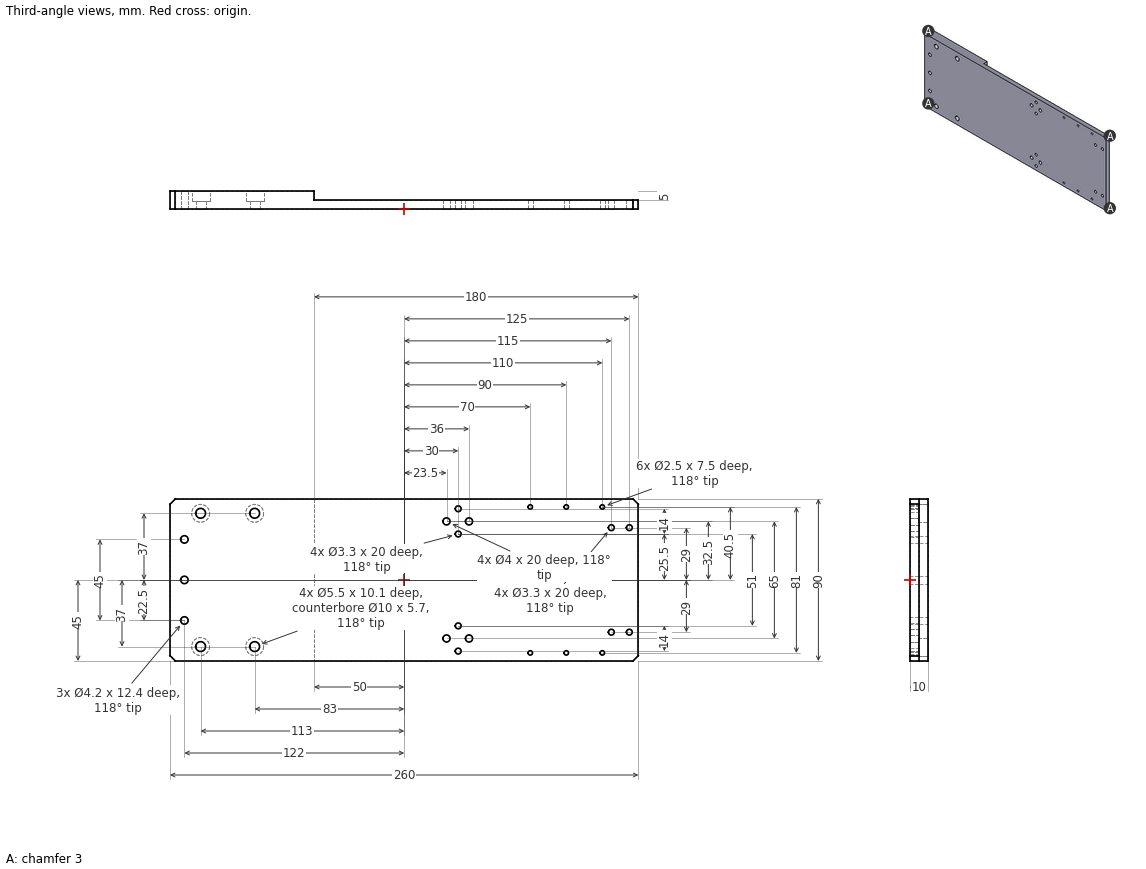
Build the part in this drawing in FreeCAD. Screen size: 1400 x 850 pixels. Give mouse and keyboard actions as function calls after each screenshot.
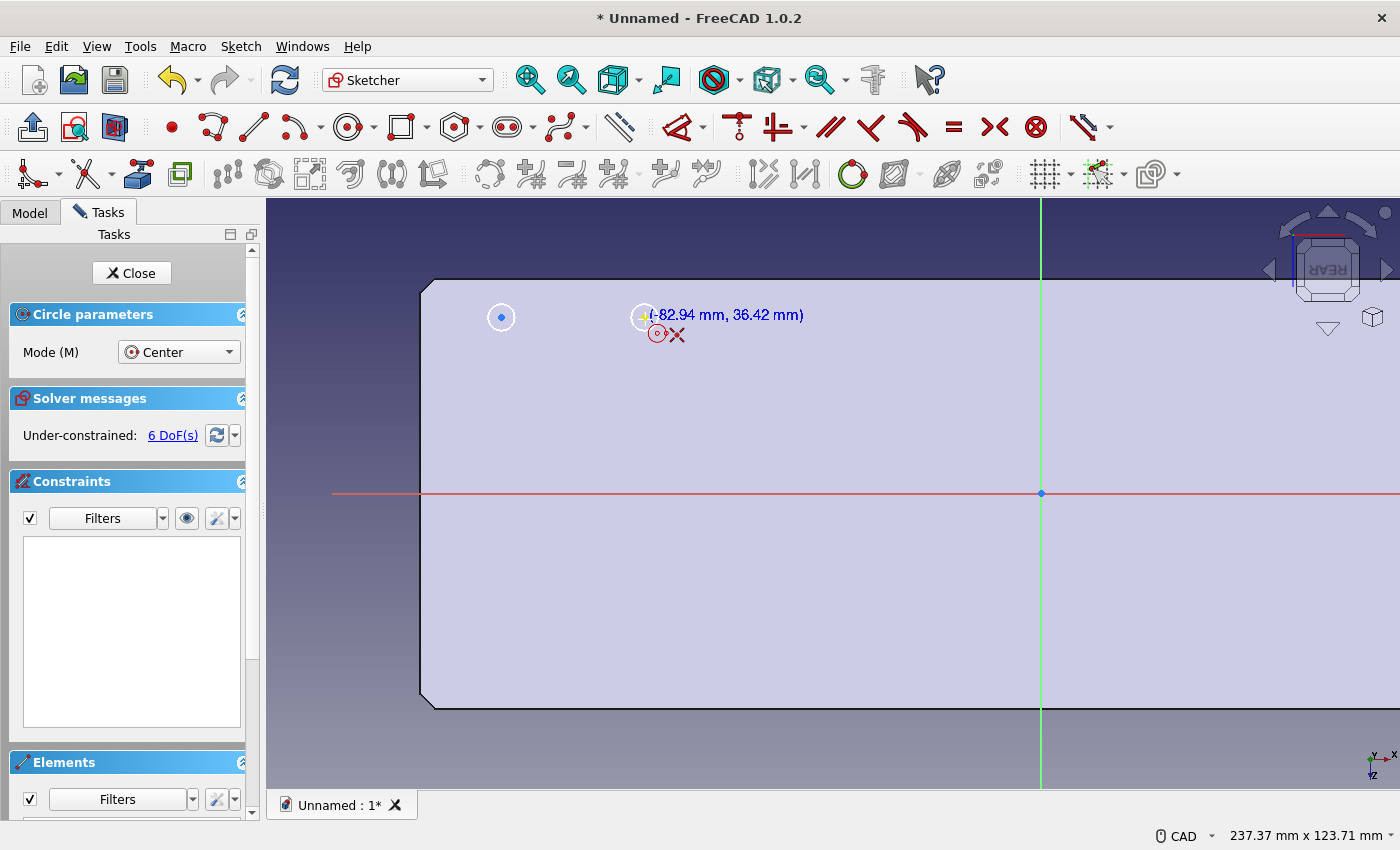
scroll(645, 670, up, 3)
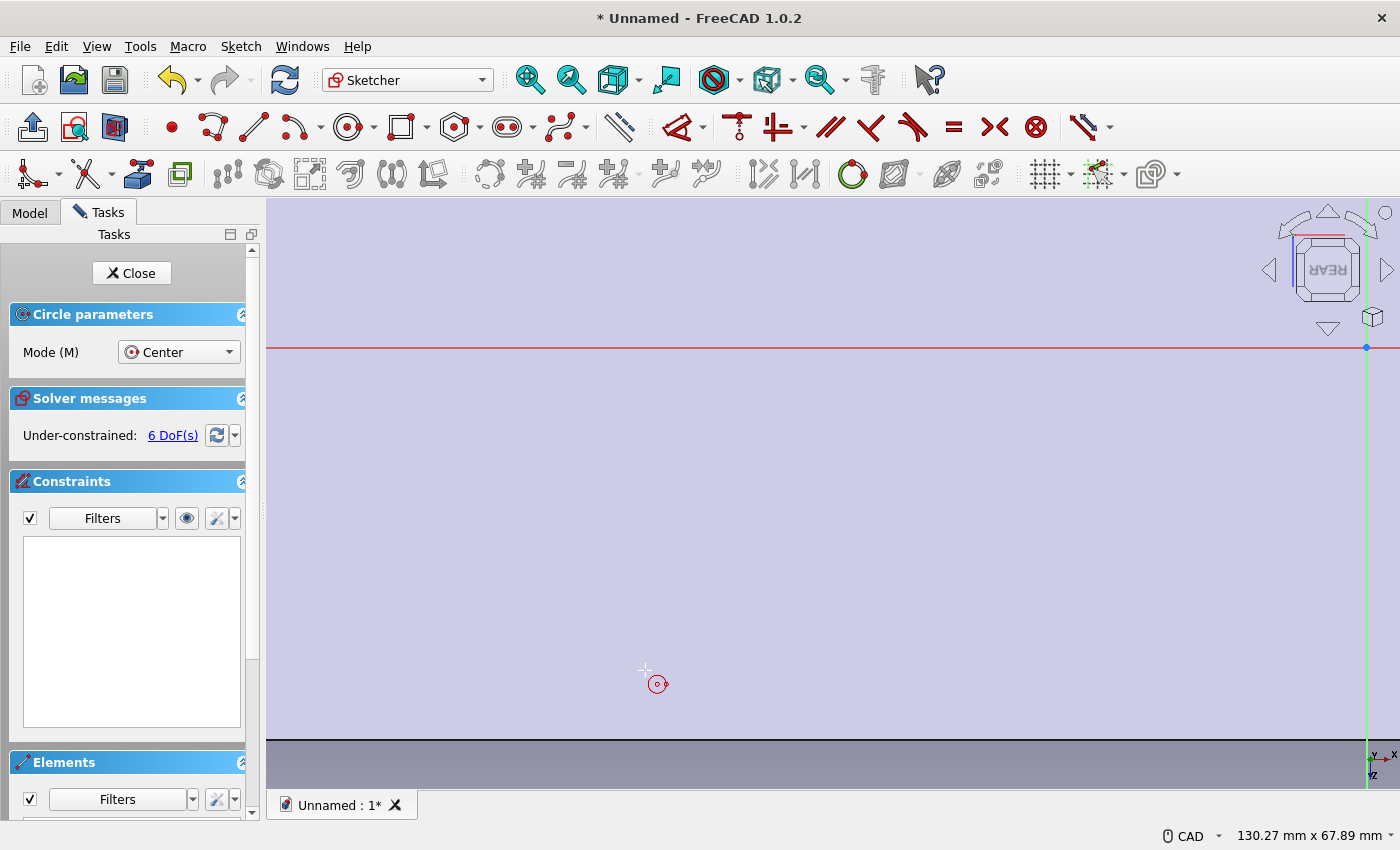
click(644, 670)
click(661, 653)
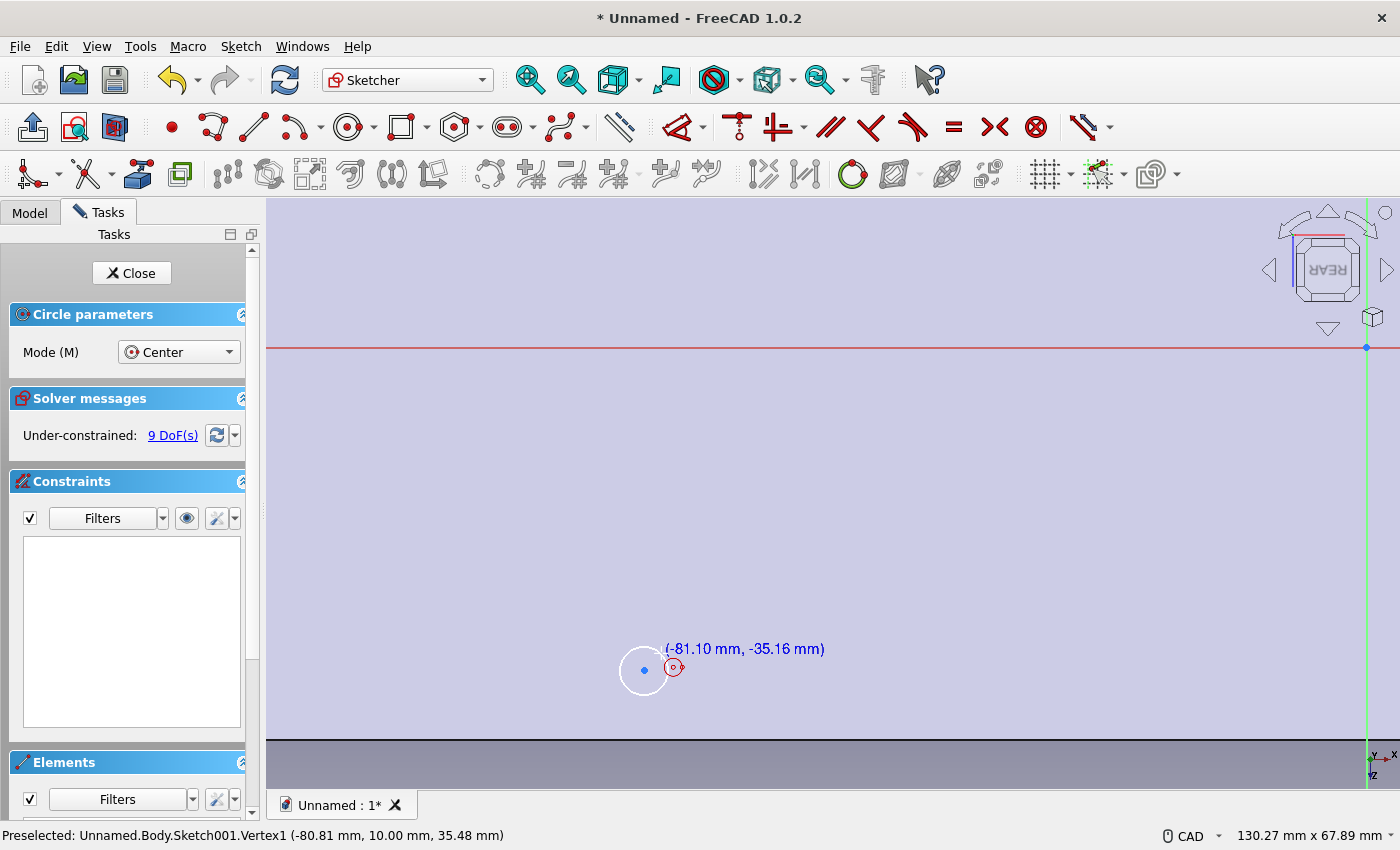
click(383, 670)
click(400, 653)
key(Escape)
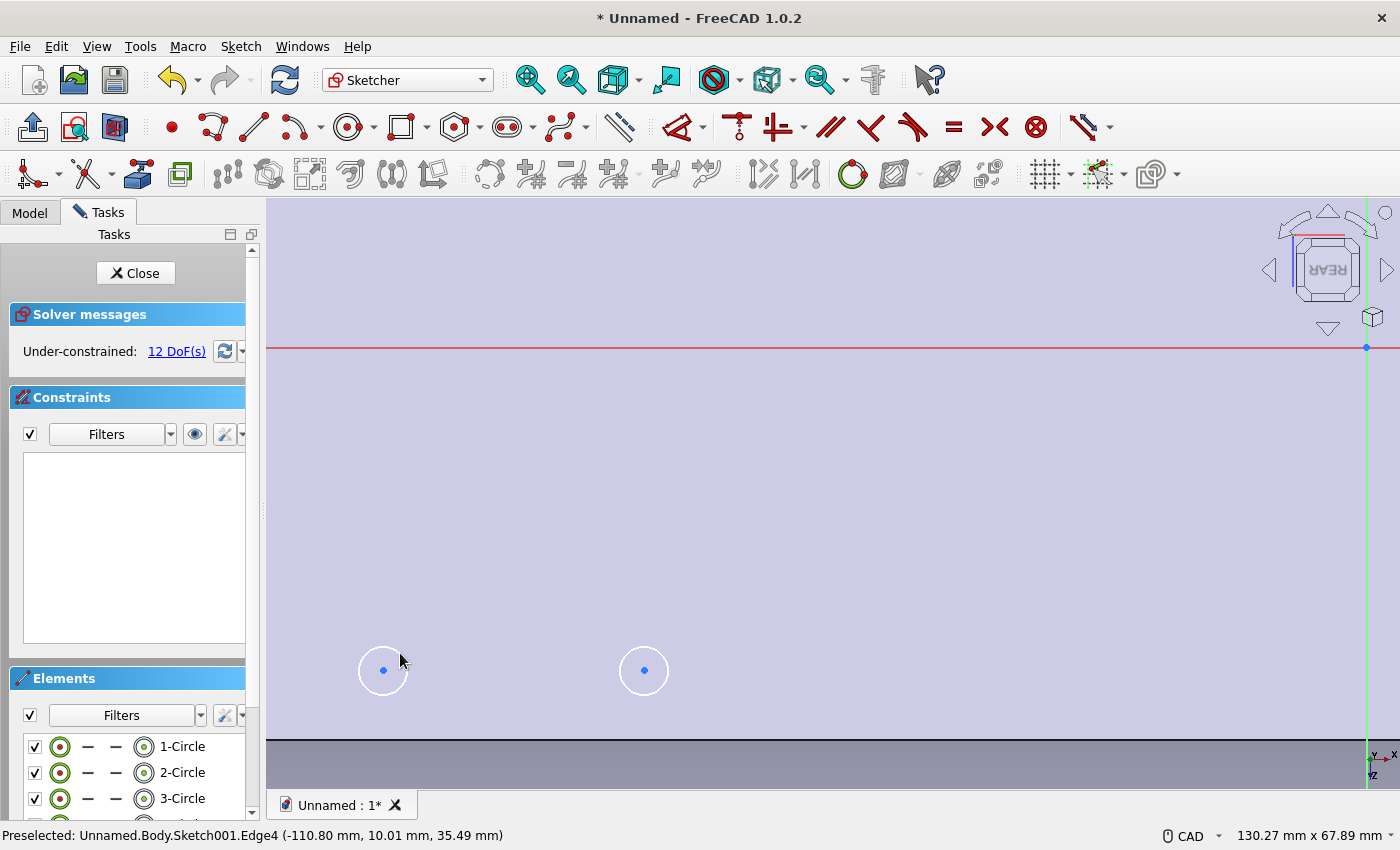
scroll(645, 671, down, 3)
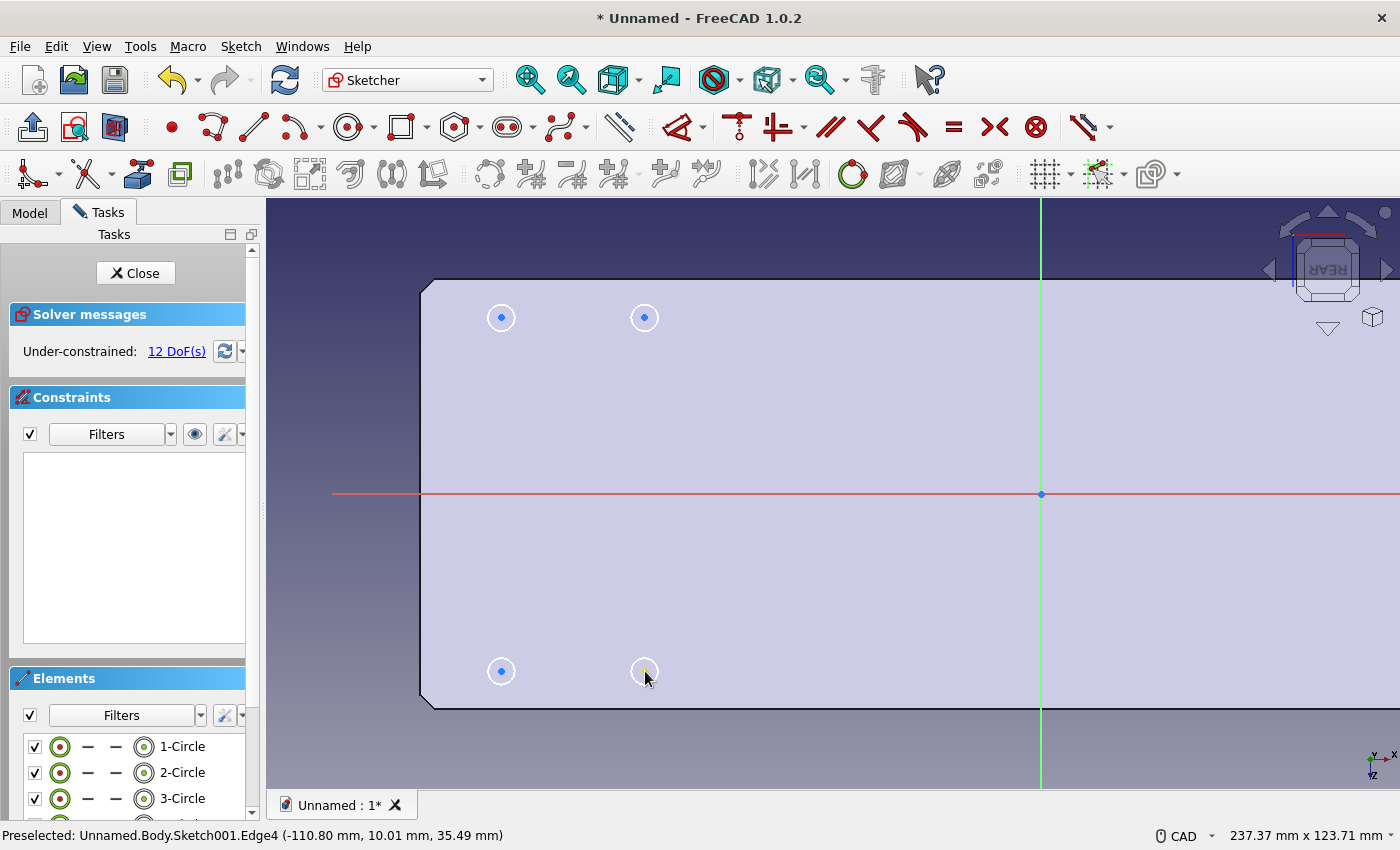
click(654, 309)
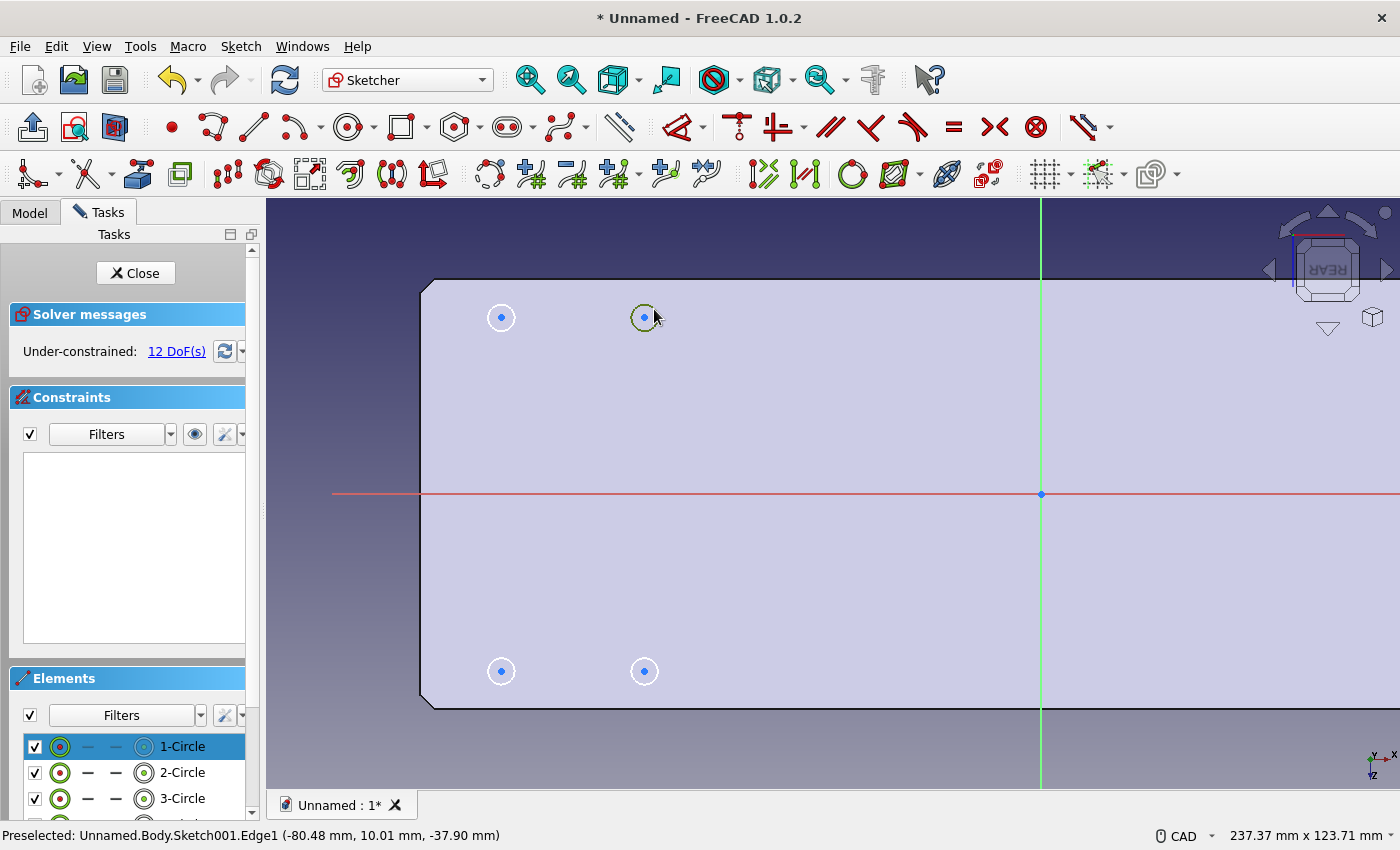
click(511, 309)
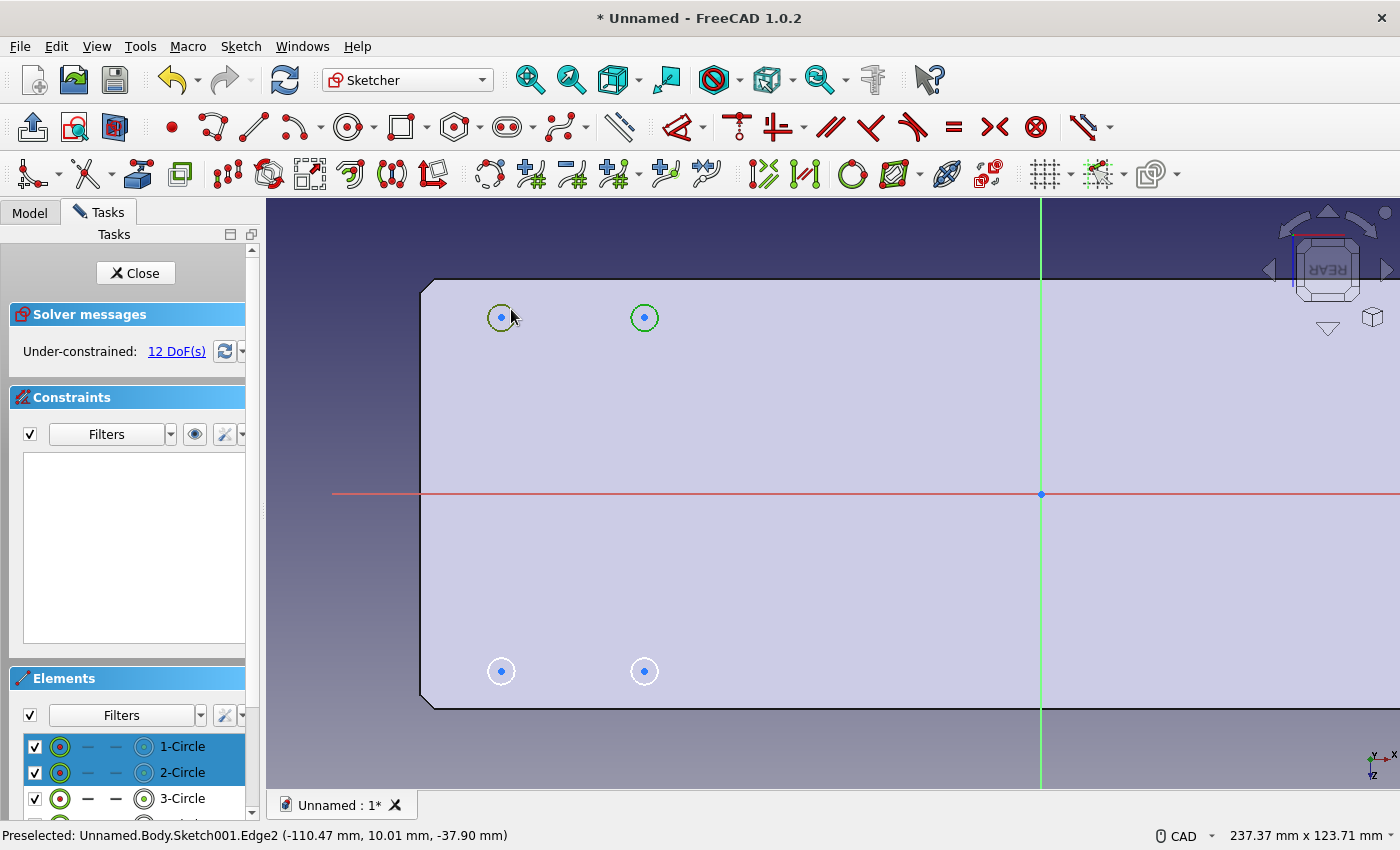
click(654, 662)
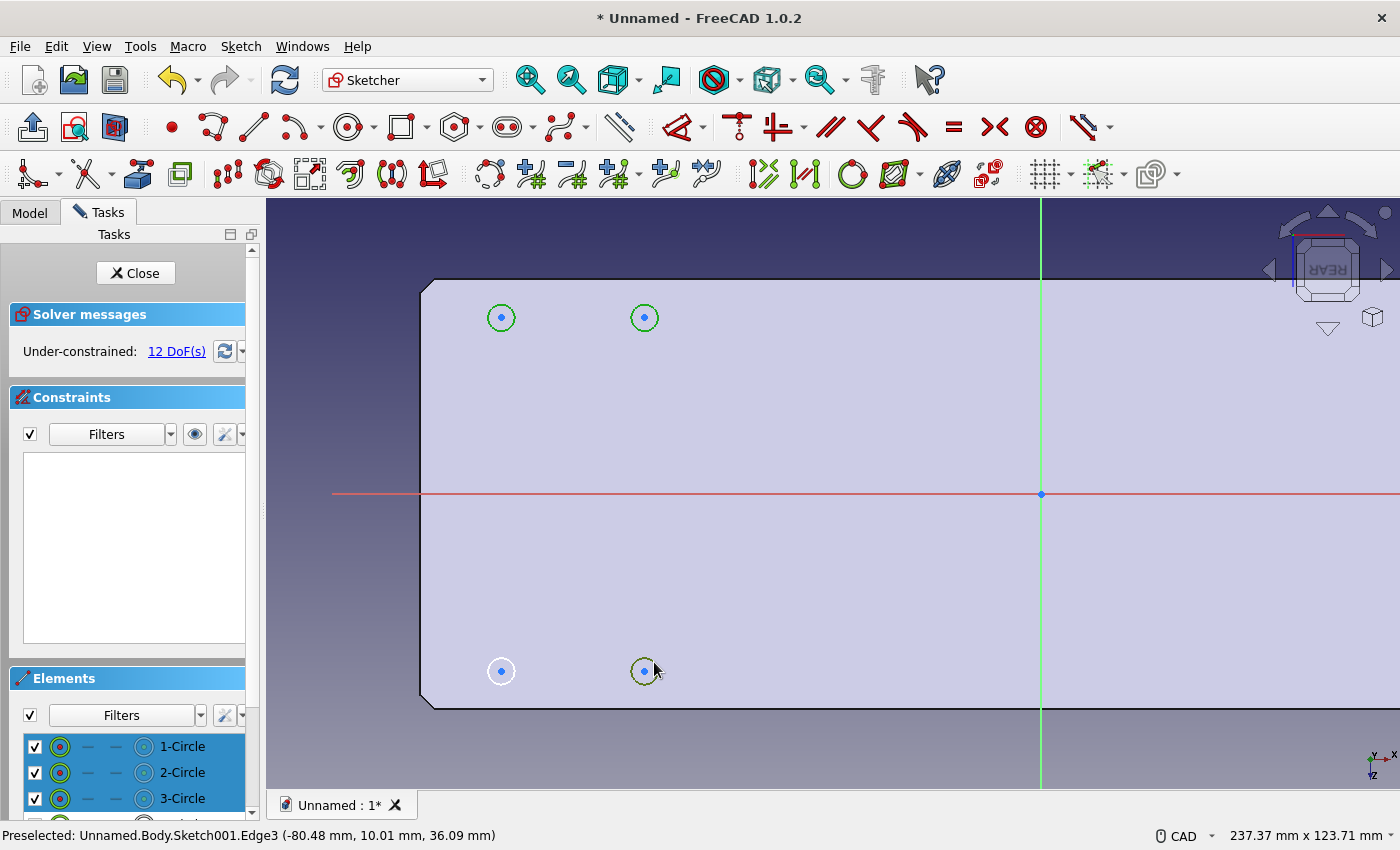
click(511, 662)